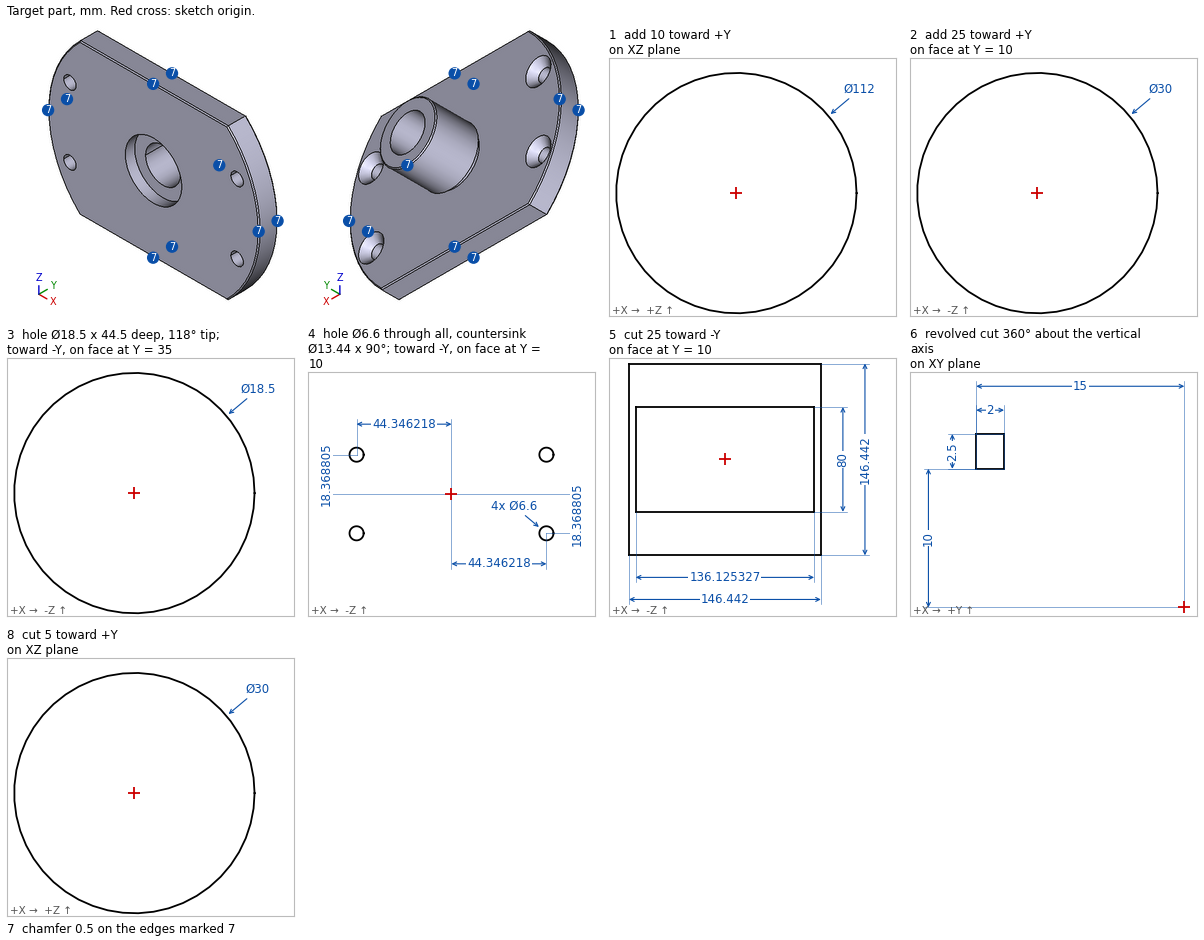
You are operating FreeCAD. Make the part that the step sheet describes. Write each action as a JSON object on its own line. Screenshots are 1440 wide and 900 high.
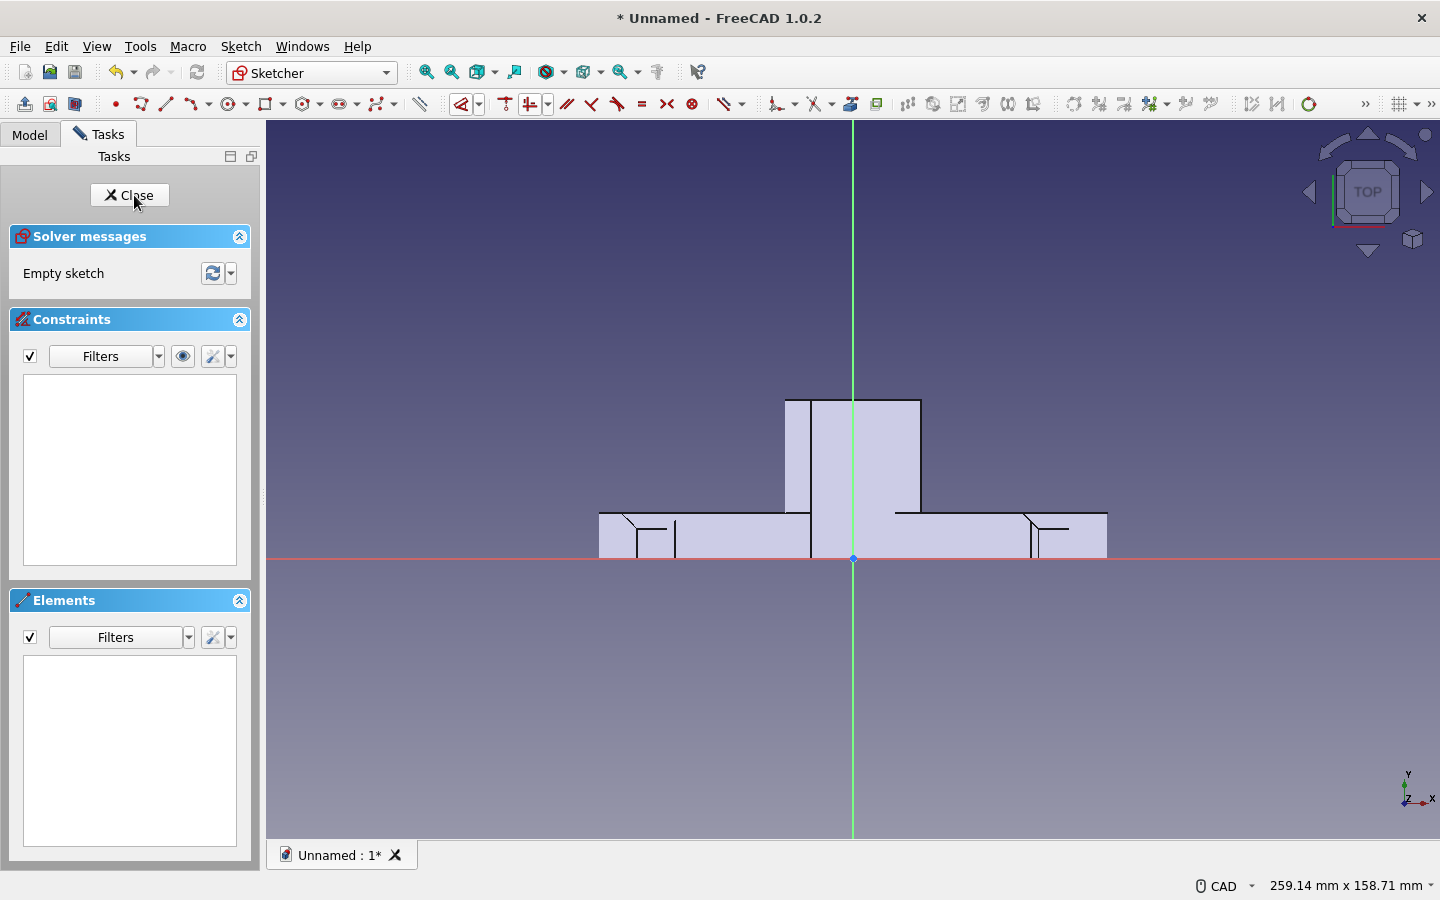
{"action": "scroll", "coordinate": [790, 509], "scroll_direction": "up", "scroll_amount": 15}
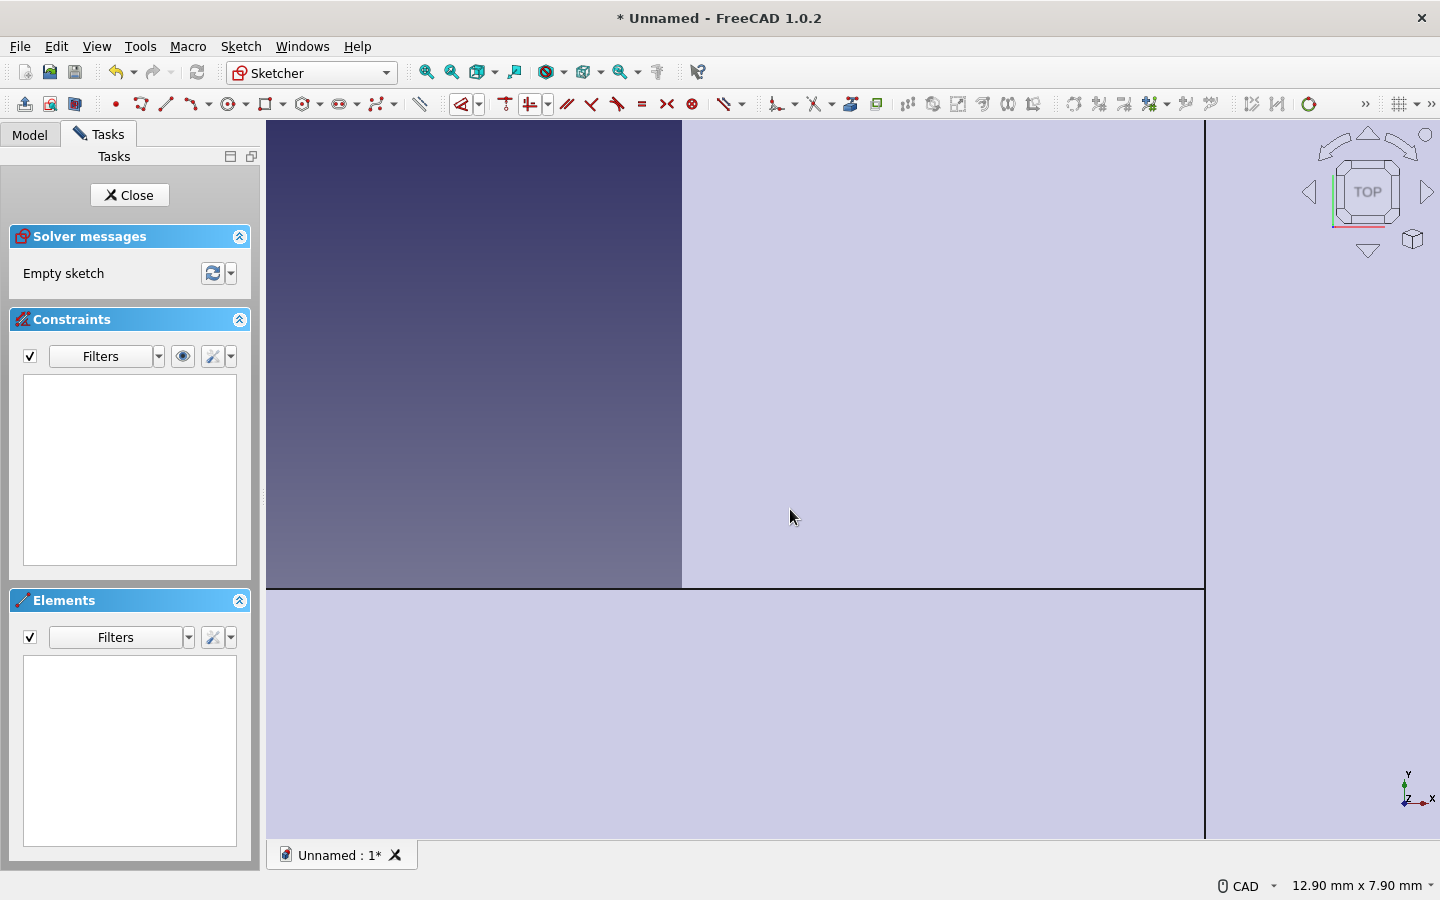
{"action": "scroll", "coordinate": [764, 471], "scroll_direction": "up", "scroll_amount": 4}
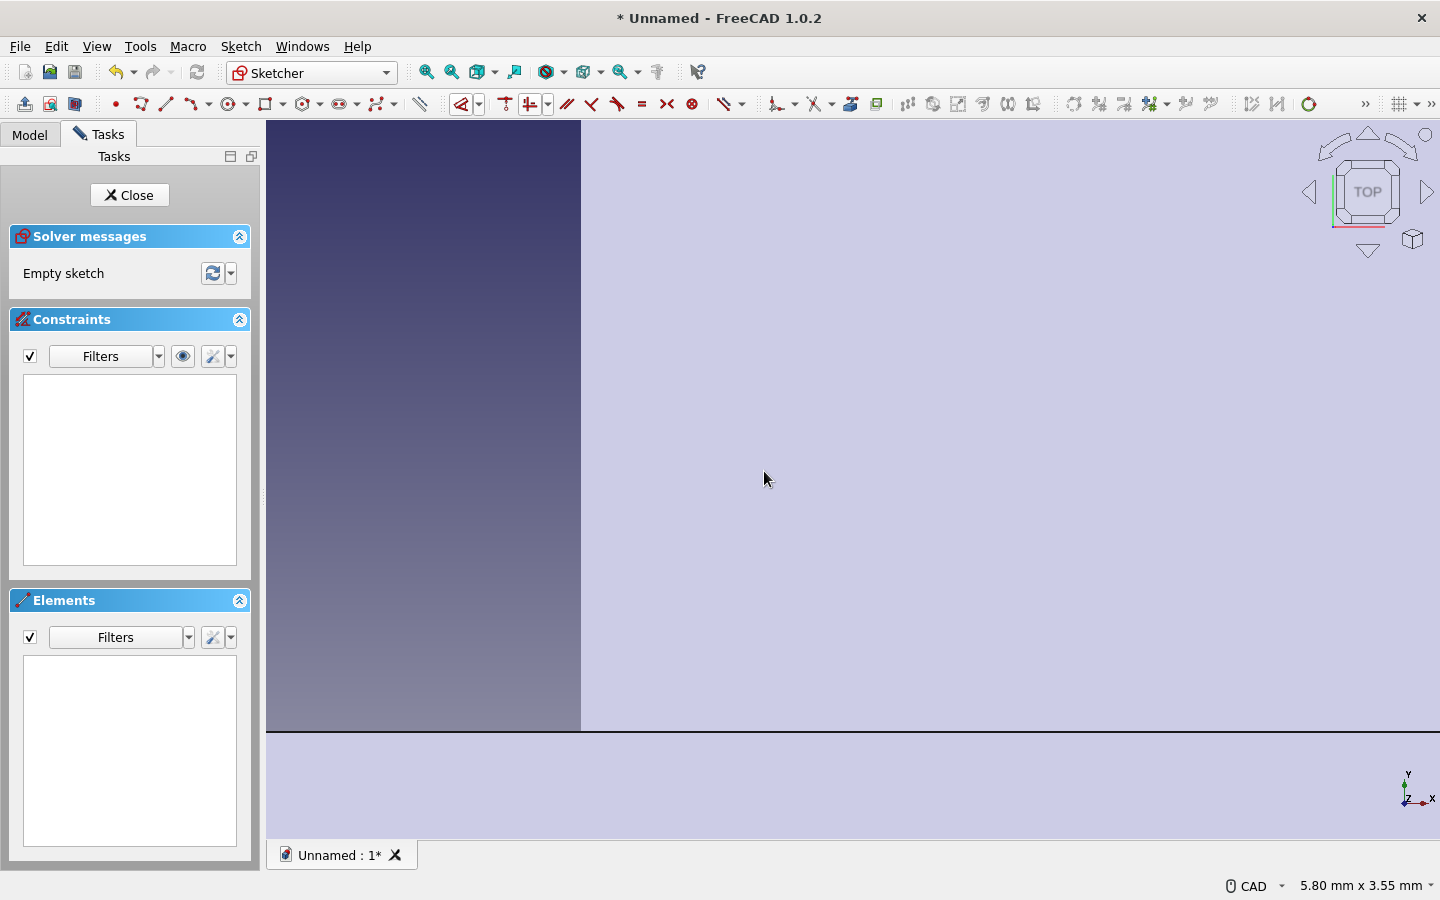
{"action": "key", "text": "g r"}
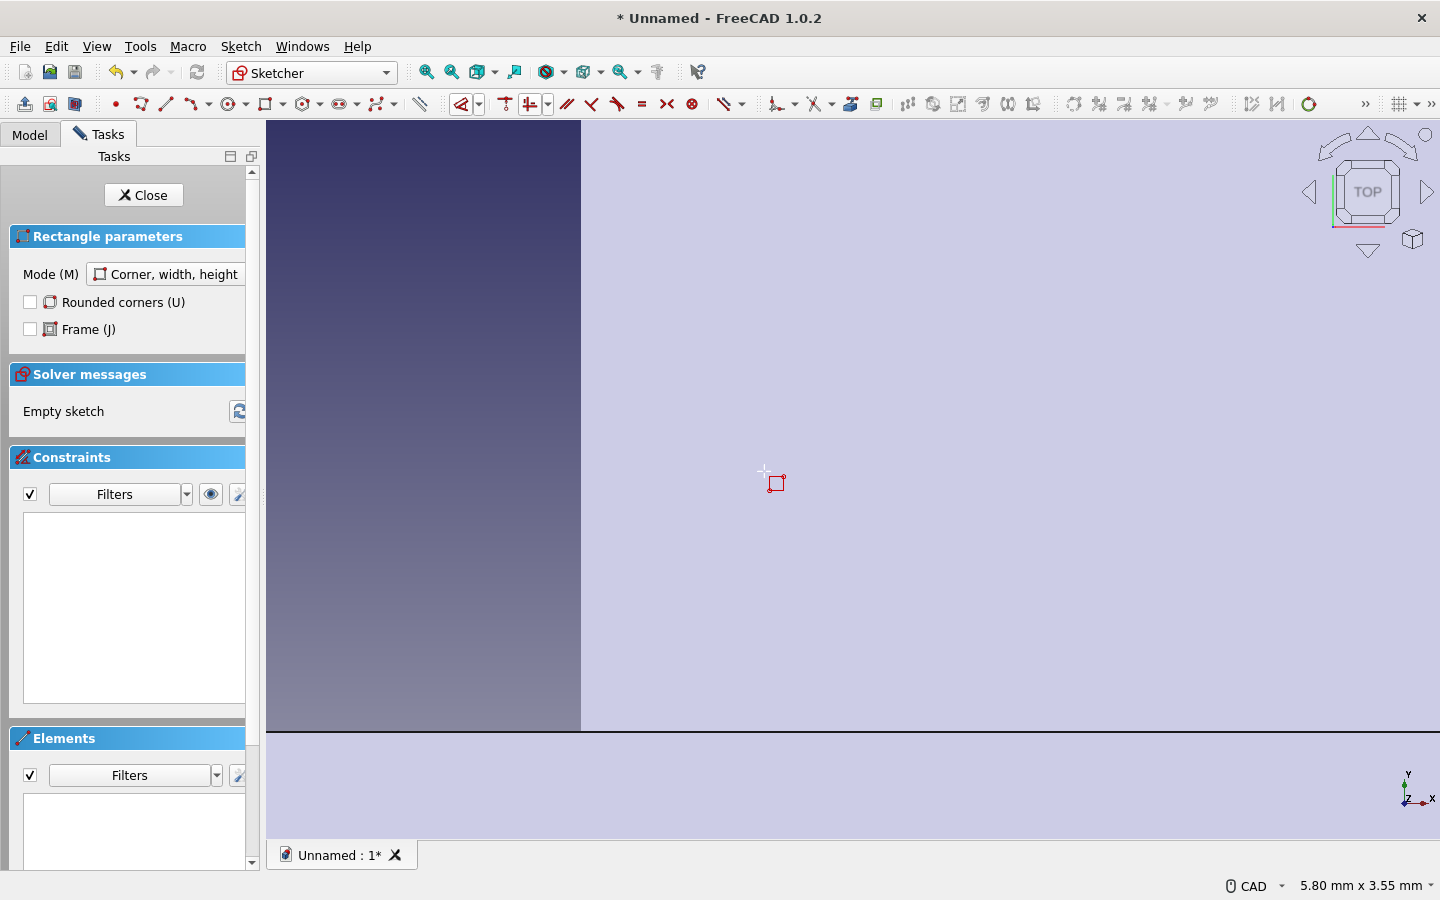
{"action": "left_click", "coordinate": [581, 226]}
{"action": "mouse_move", "coordinate": [986, 732]}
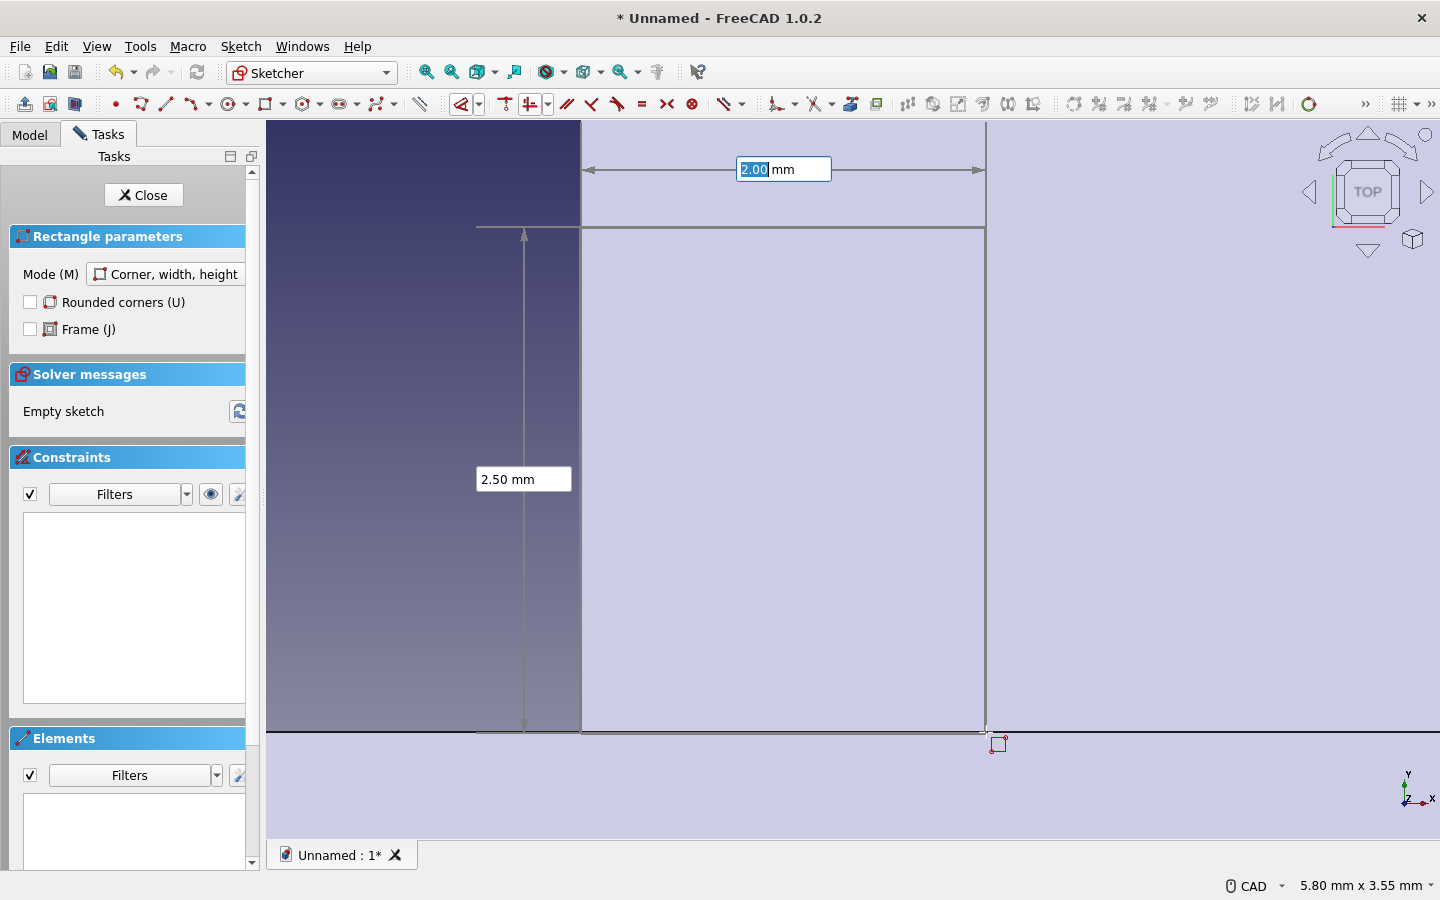
{"action": "type", "text": "2"}
{"action": "key", "text": "Tab"}
{"action": "type", "text": "2.5"}
{"action": "key", "text": "Return"}
{"action": "key", "text": "Escape"}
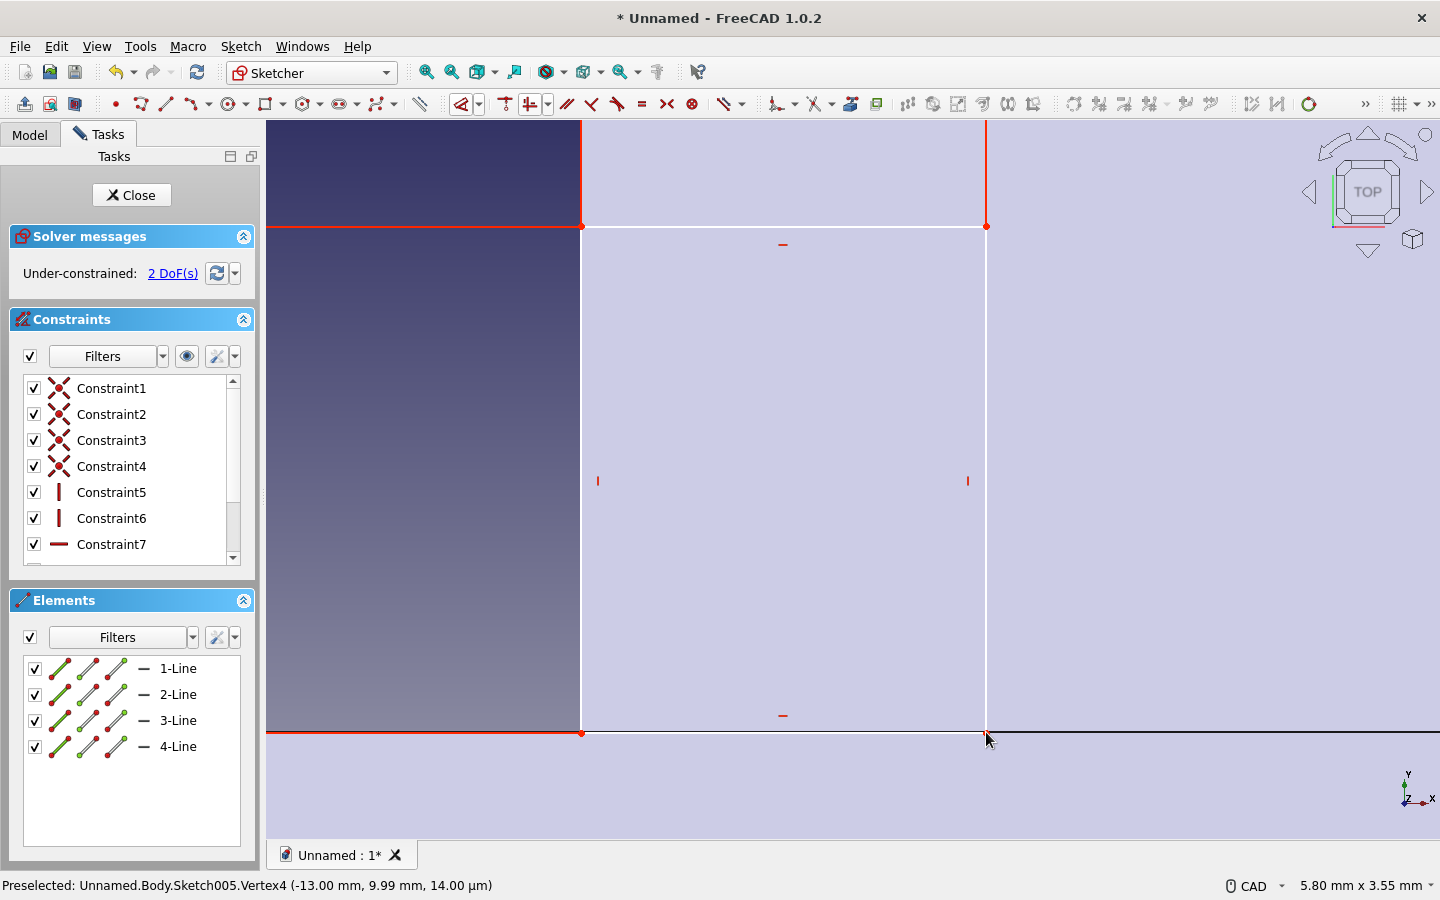
{"action": "left_click", "coordinate": [581, 227]}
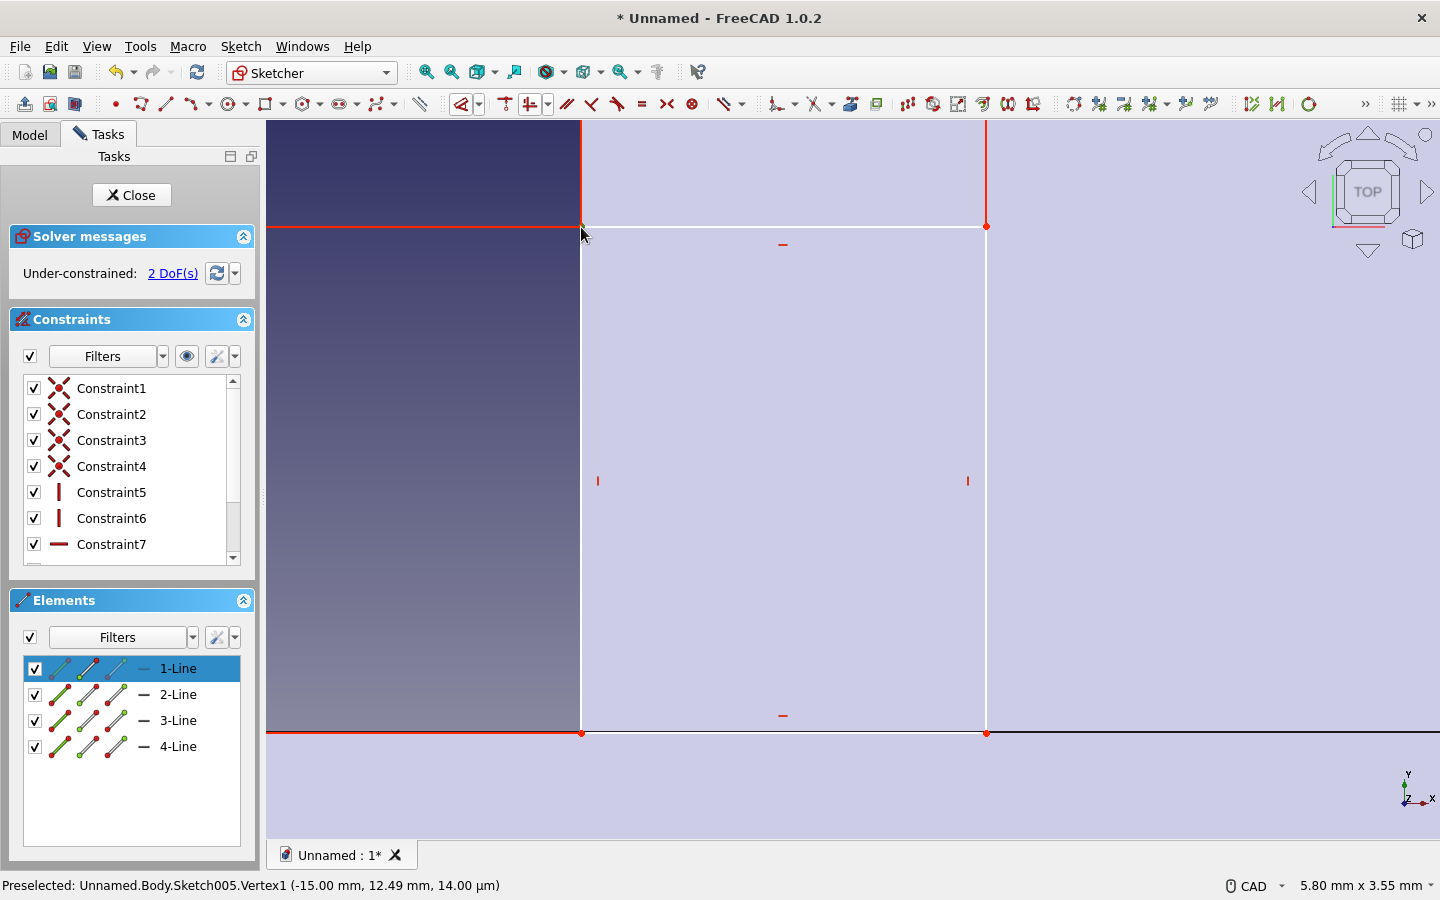
{"action": "key", "text": "l"}